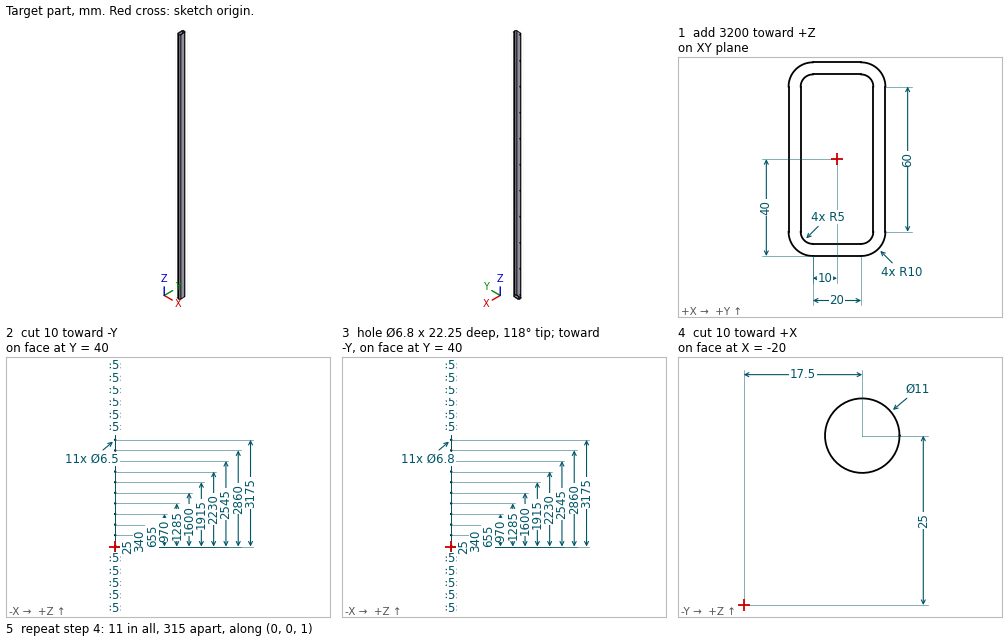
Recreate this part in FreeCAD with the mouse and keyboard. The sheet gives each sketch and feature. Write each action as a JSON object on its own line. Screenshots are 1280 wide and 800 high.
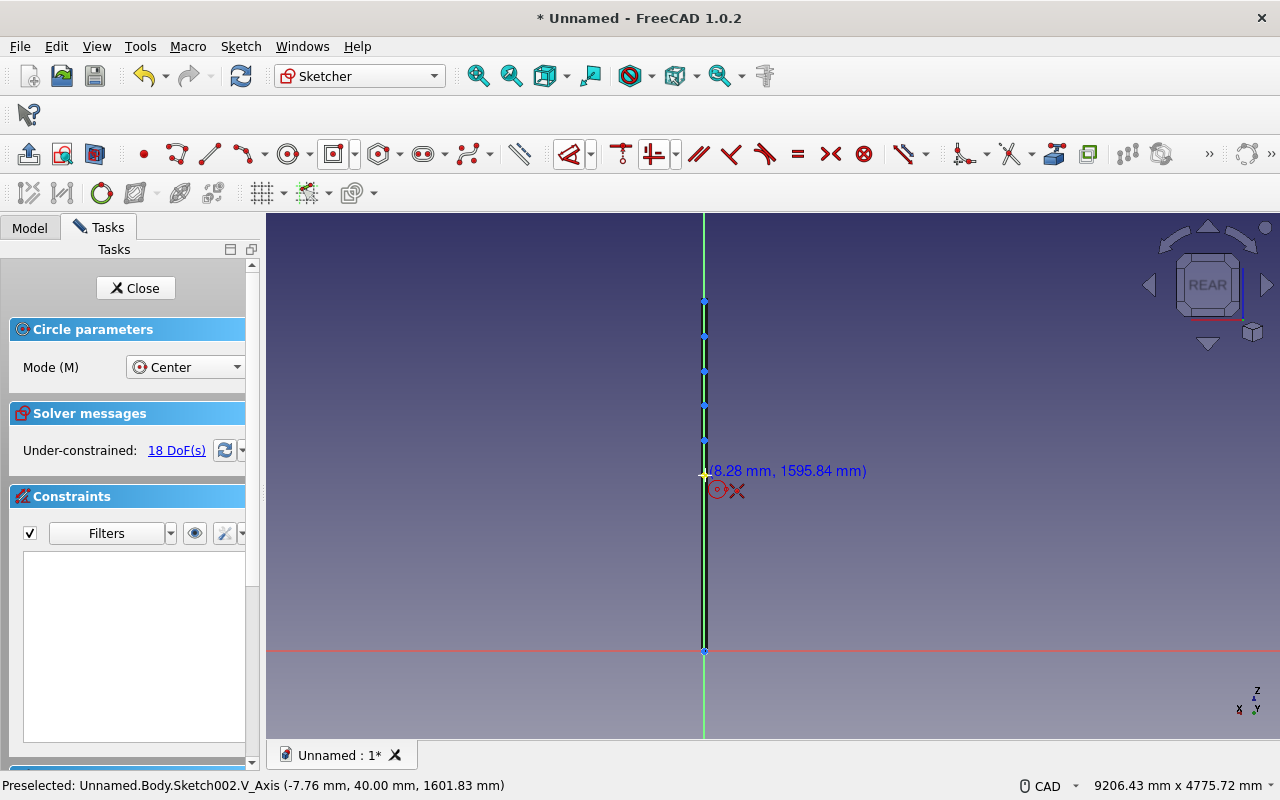
{"action": "scroll", "coordinate": [705, 510], "scroll_direction": "up", "scroll_amount": 21}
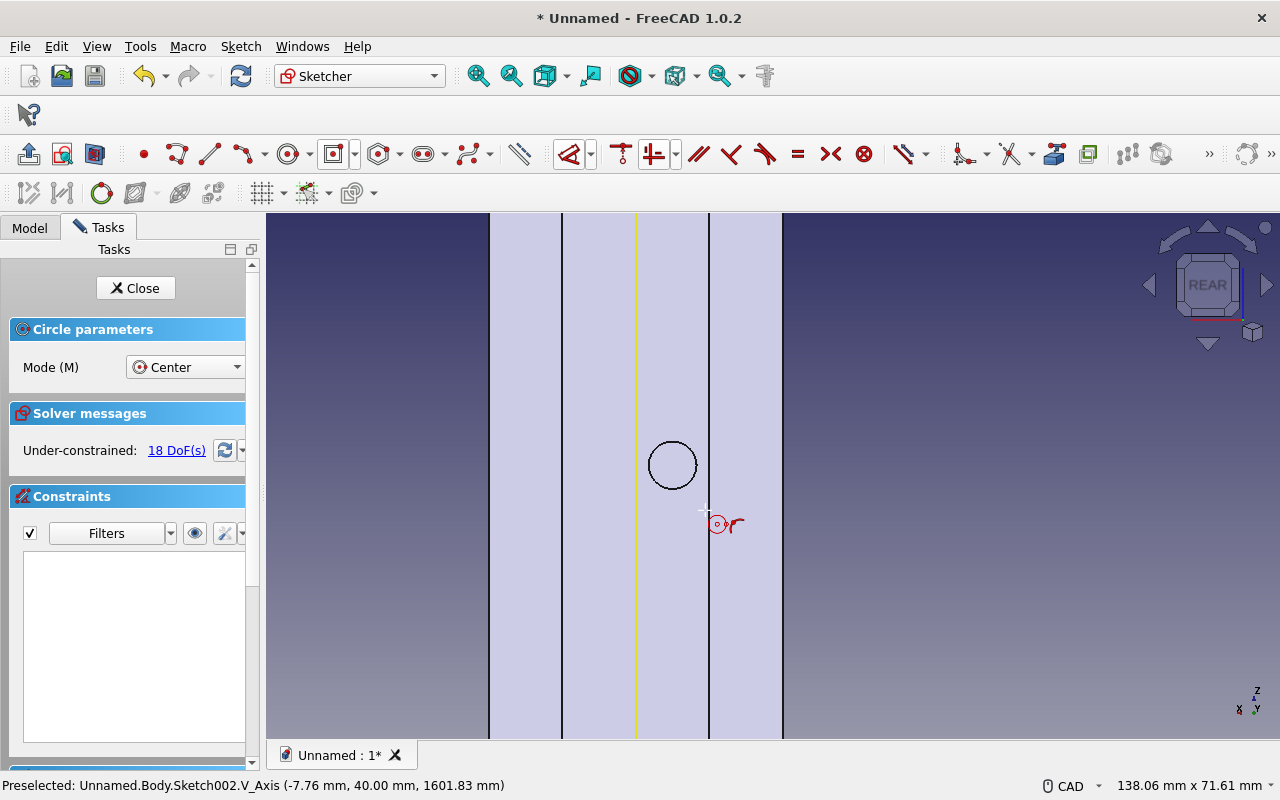
{"action": "left_click", "coordinate": [673, 465]}
{"action": "left_click", "coordinate": [690, 448]}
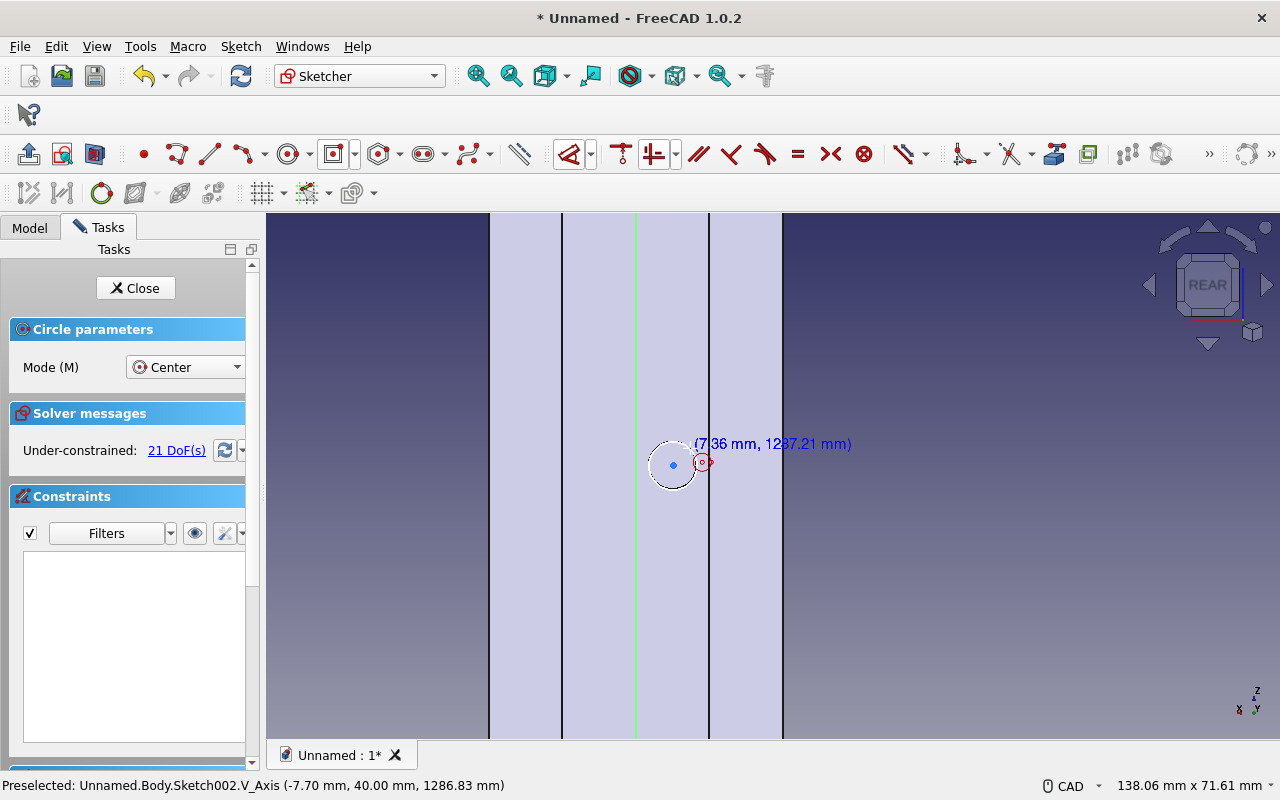
{"action": "scroll", "coordinate": [704, 476], "scroll_direction": "down", "scroll_amount": 15}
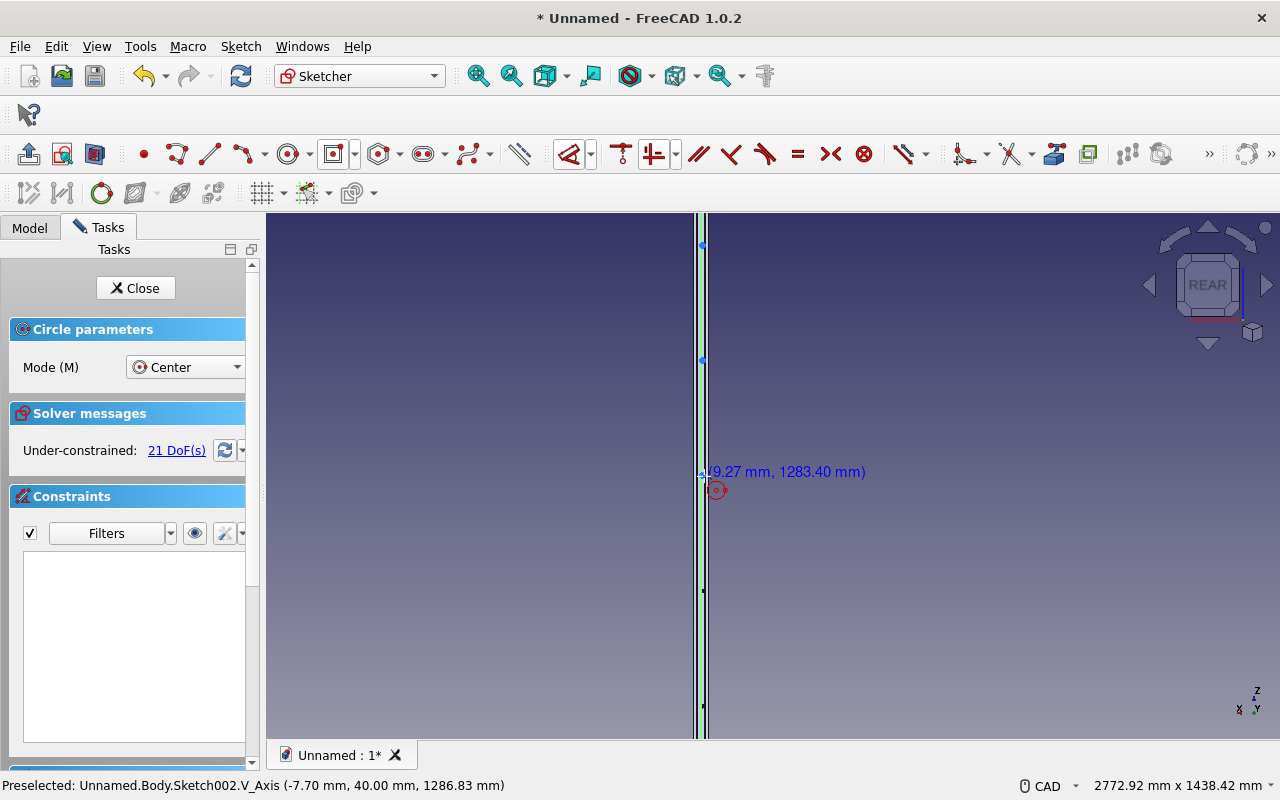
{"action": "scroll", "coordinate": [705, 524], "scroll_direction": "down", "scroll_amount": 6}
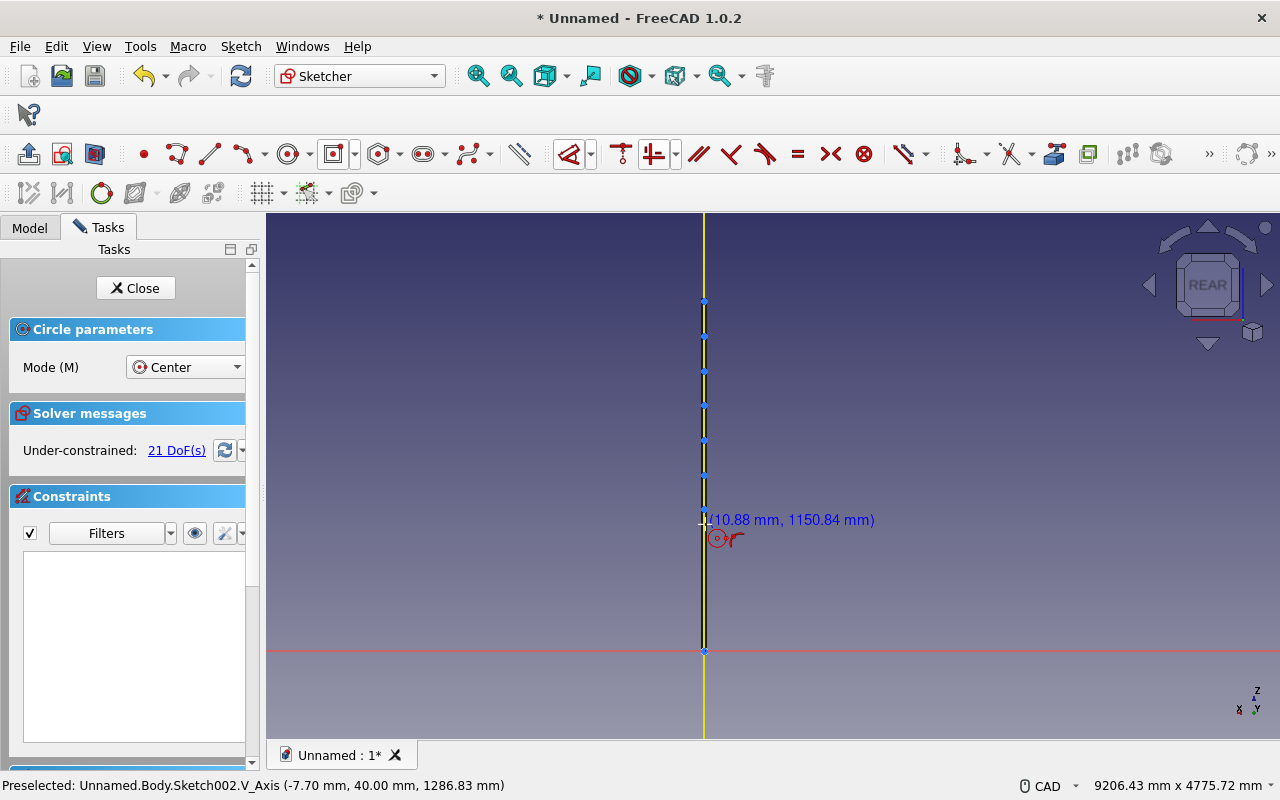
{"action": "scroll", "coordinate": [705, 545], "scroll_direction": "up", "scroll_amount": 21}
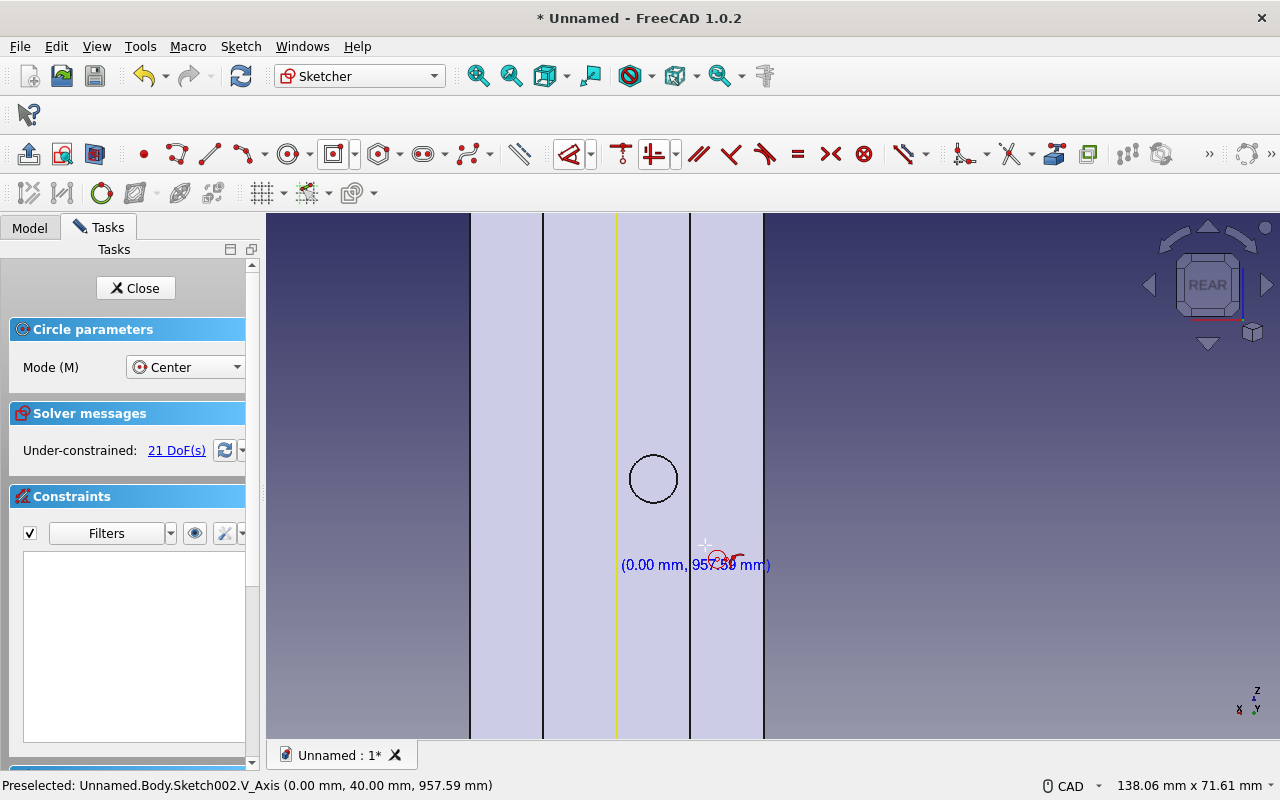
{"action": "left_click", "coordinate": [654, 479]}
{"action": "left_click", "coordinate": [671, 461]}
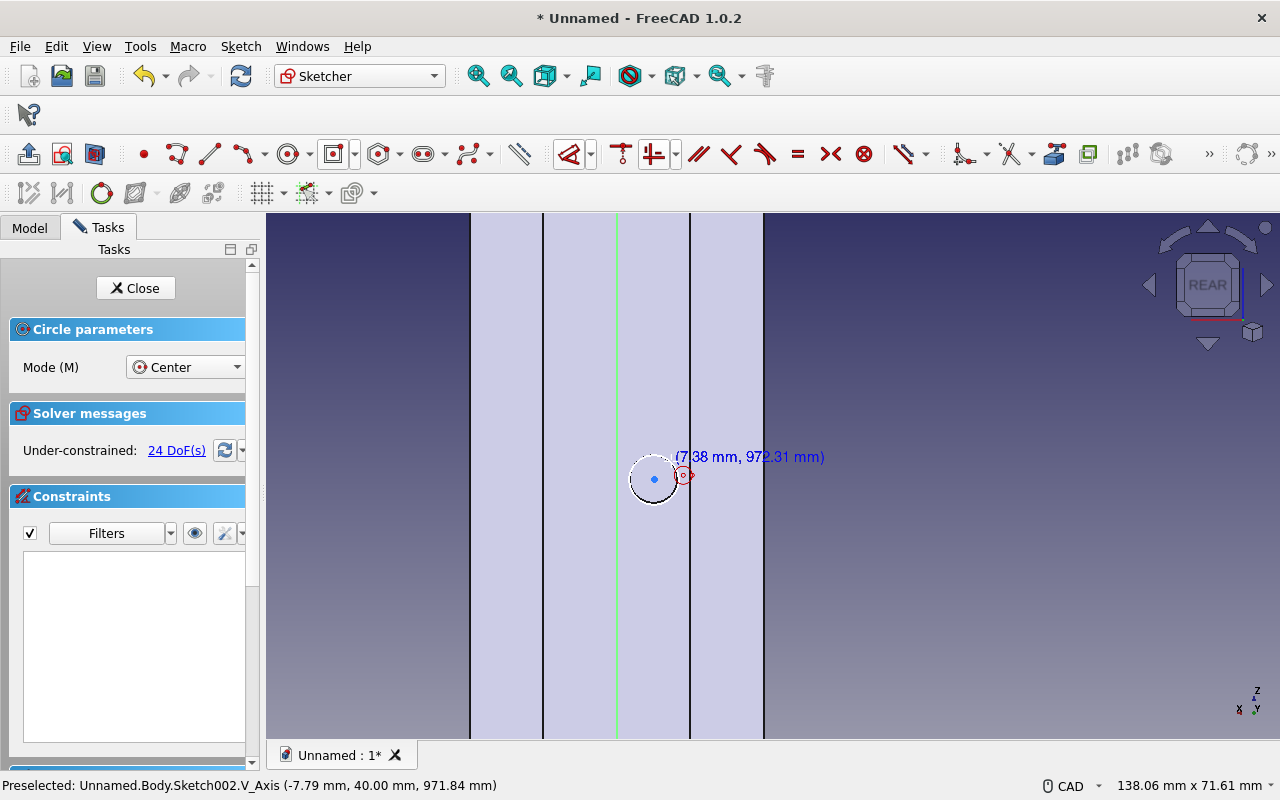
{"action": "scroll", "coordinate": [704, 476], "scroll_direction": "down", "scroll_amount": 15}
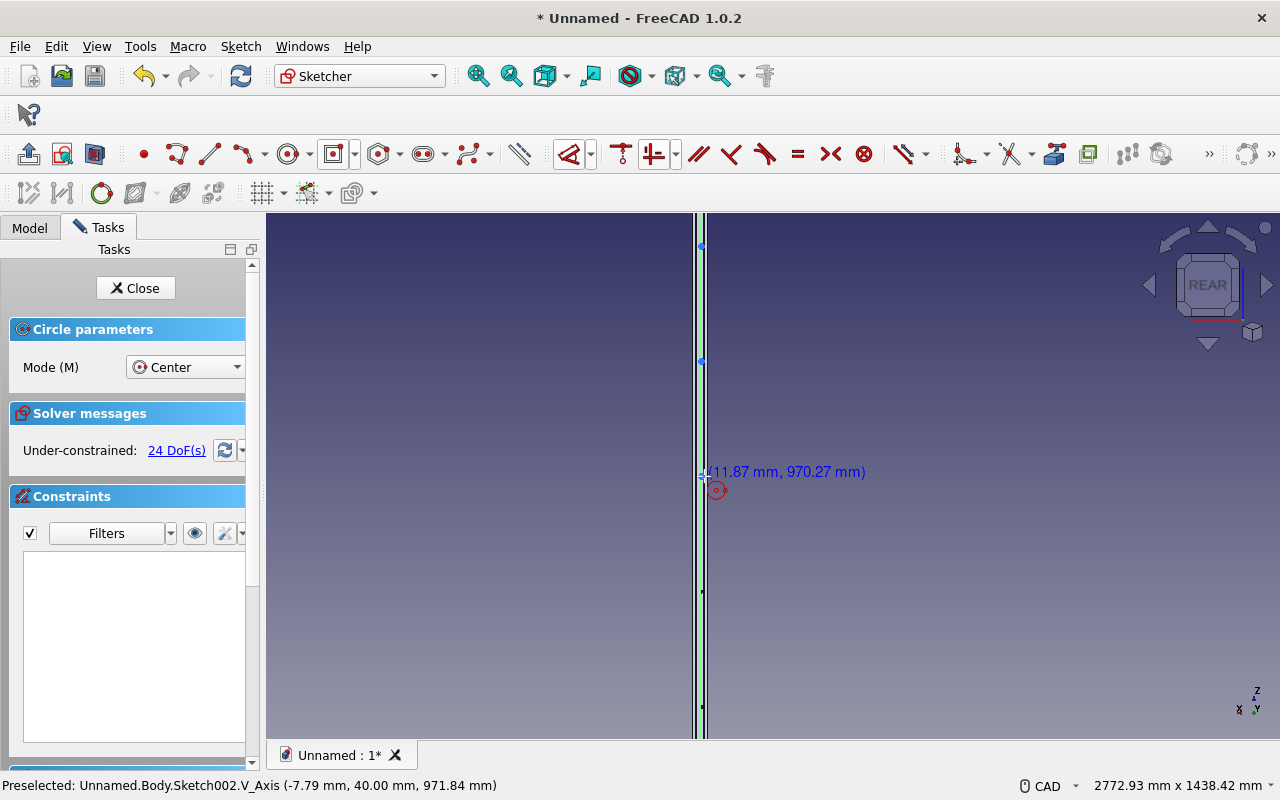
{"action": "scroll", "coordinate": [706, 573], "scroll_direction": "down", "scroll_amount": 6}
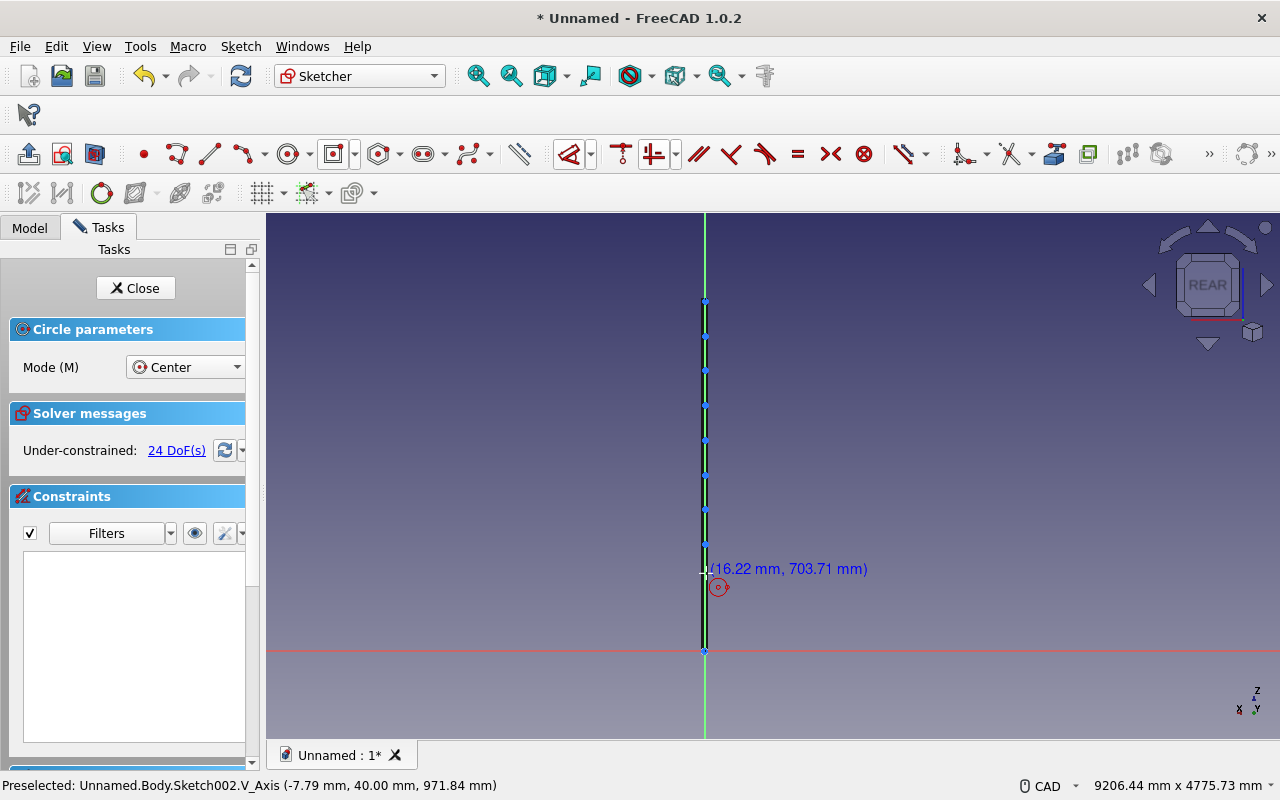
{"action": "scroll", "coordinate": [705, 579], "scroll_direction": "up", "scroll_amount": 21}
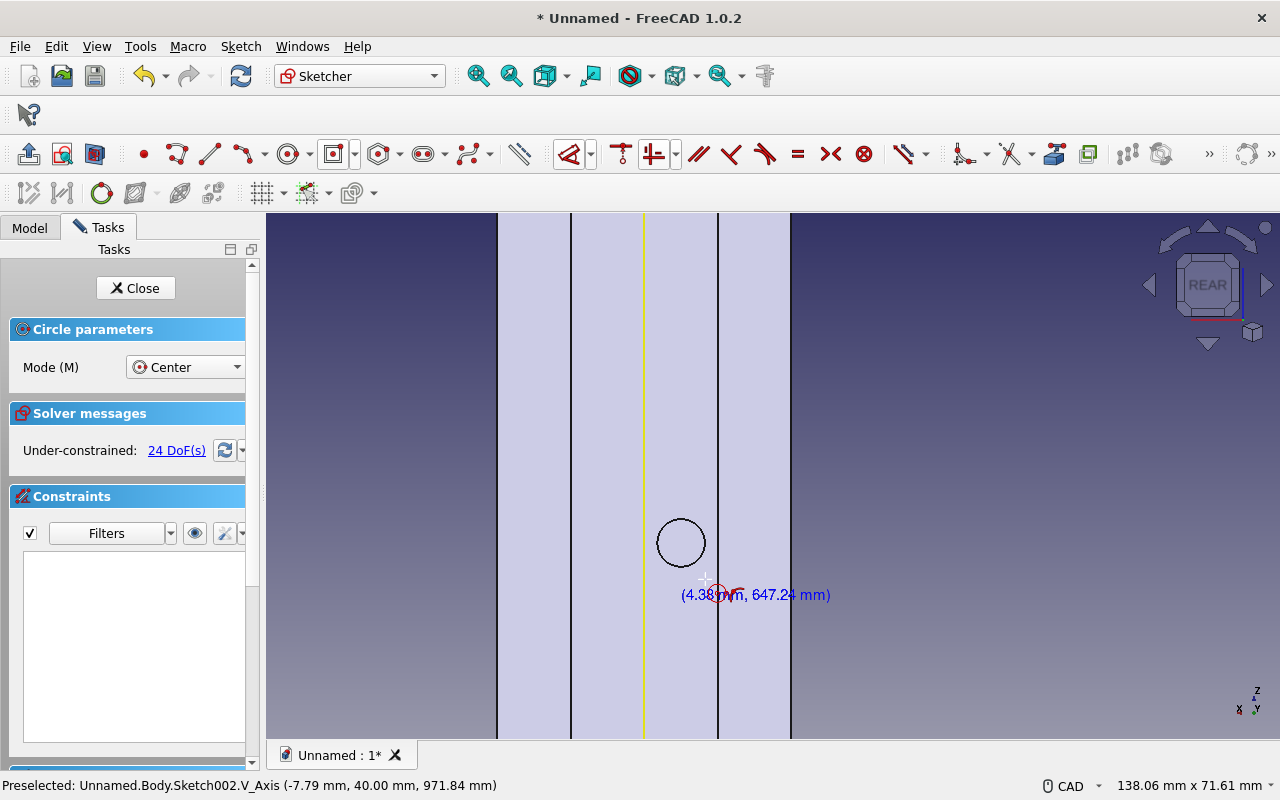
{"action": "left_click", "coordinate": [681, 543]}
{"action": "left_click", "coordinate": [699, 525]}